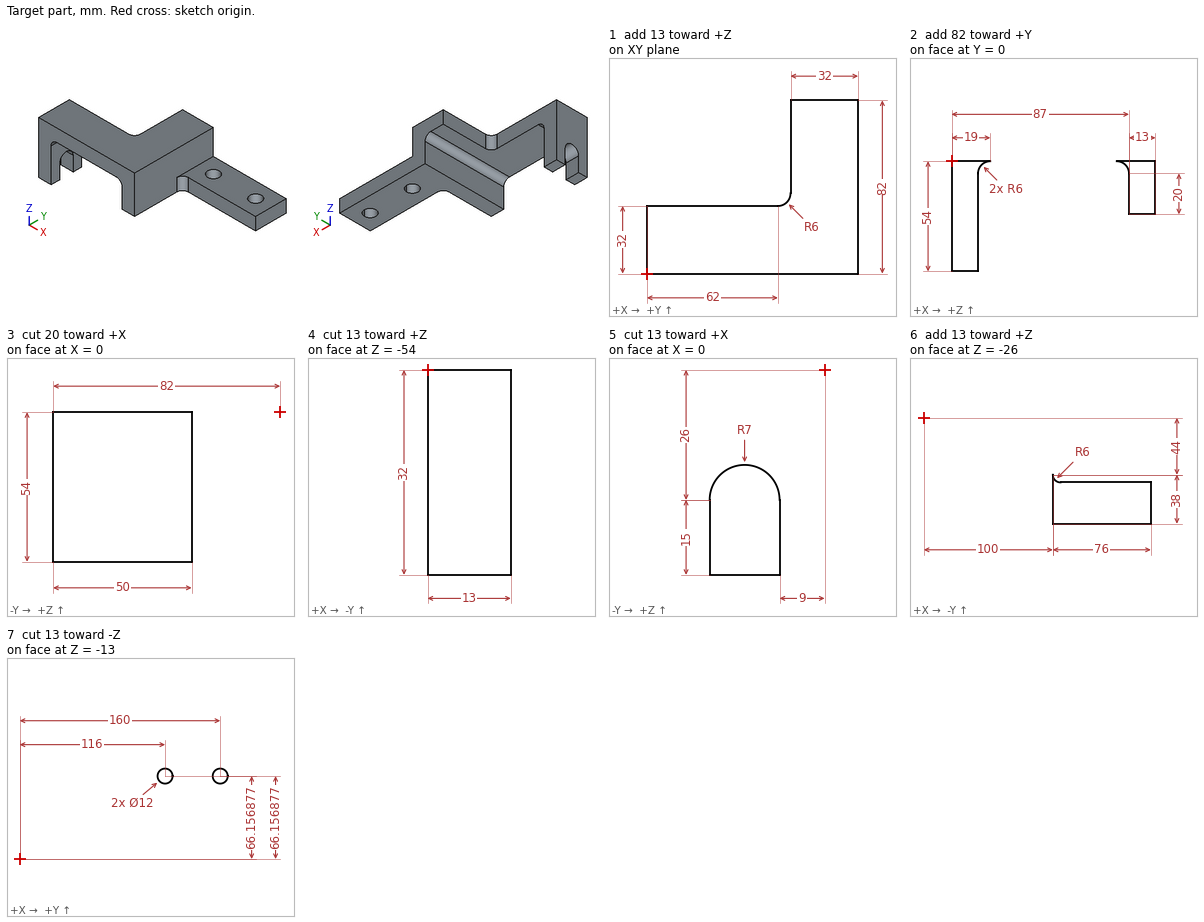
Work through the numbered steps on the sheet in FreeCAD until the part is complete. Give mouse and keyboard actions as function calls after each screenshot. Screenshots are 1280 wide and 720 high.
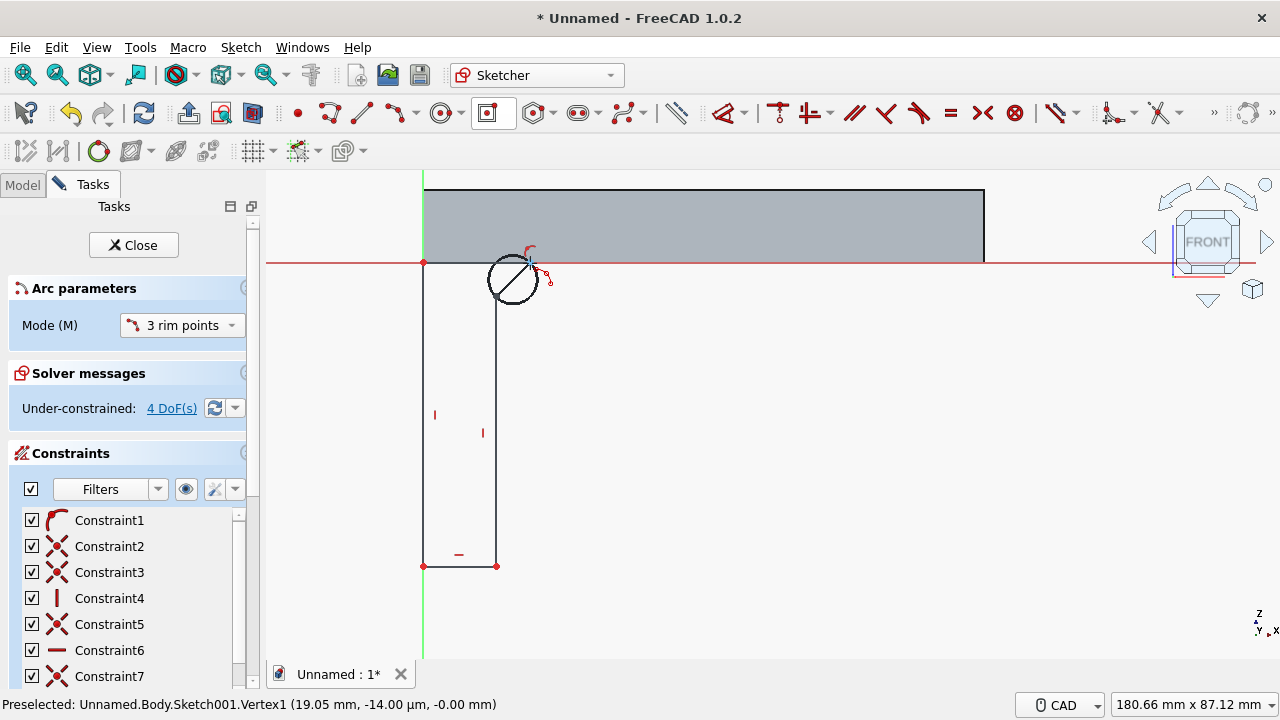
scroll(506, 272, up, 3)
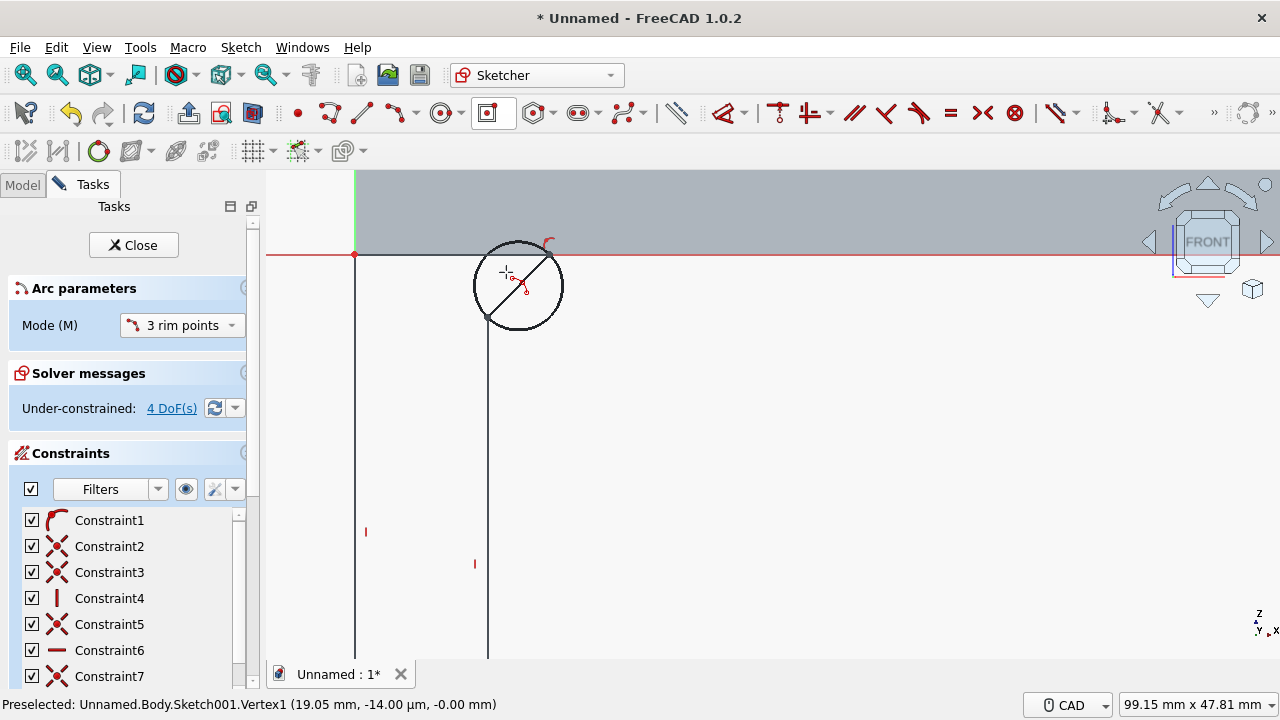
click(506, 273)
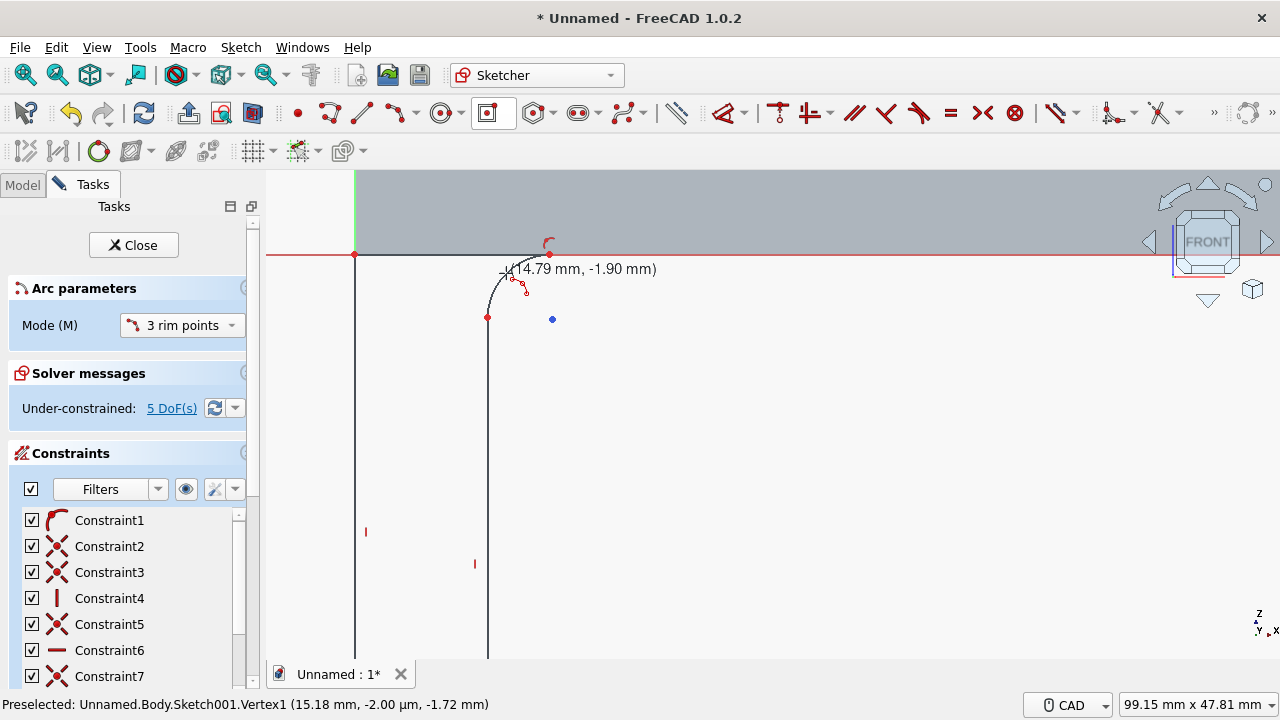
click(330, 114)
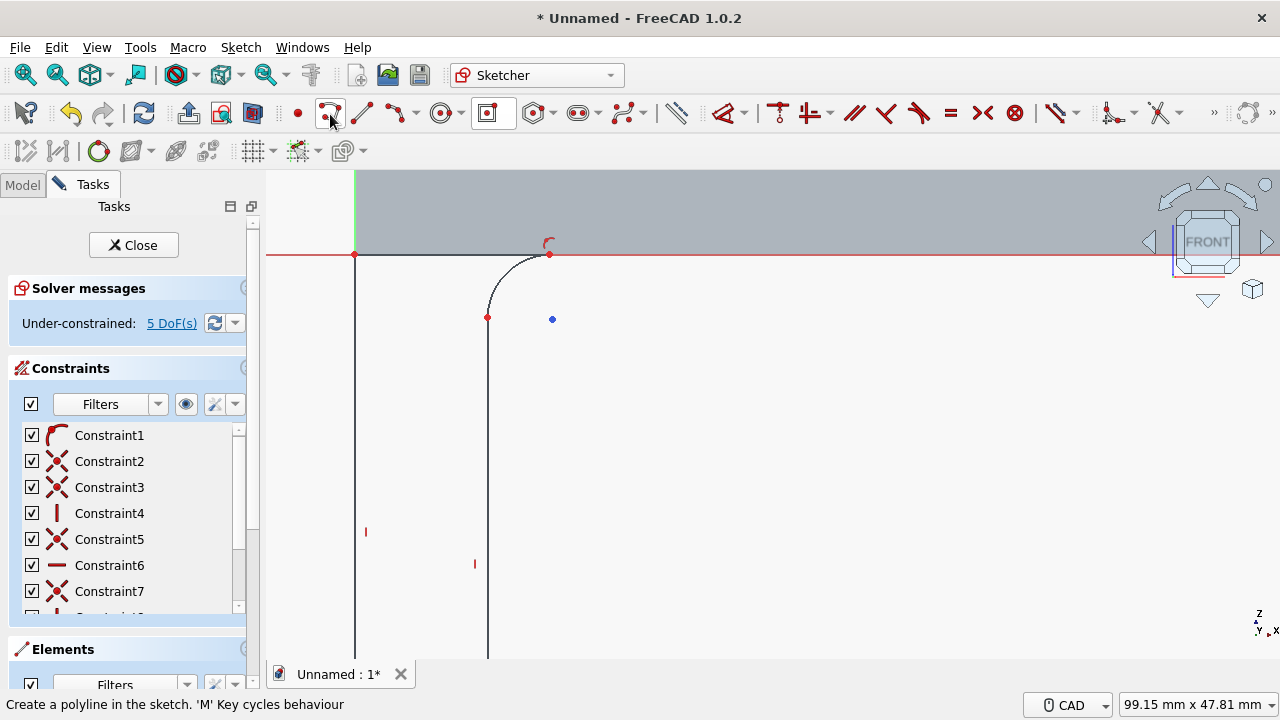
scroll(508, 273, down, 3)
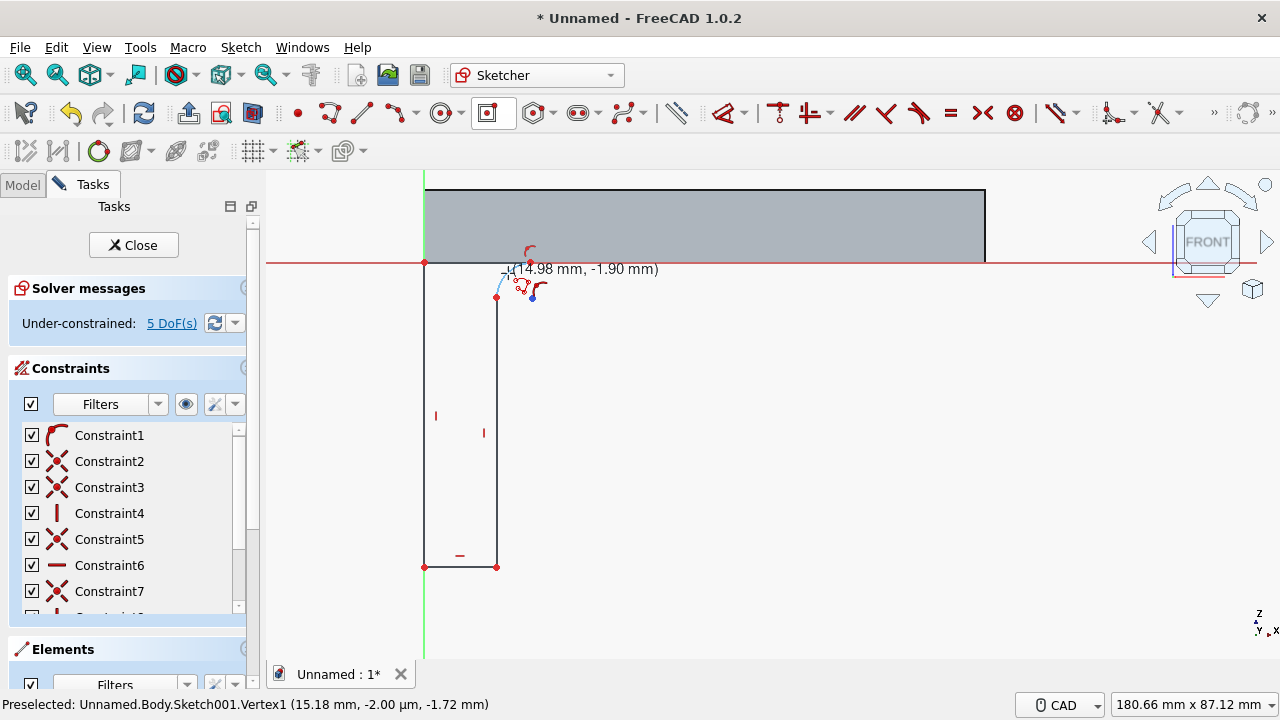
click(912, 297)
click(912, 409)
click(985, 409)
click(985, 263)
click(879, 272)
right_click(879, 272)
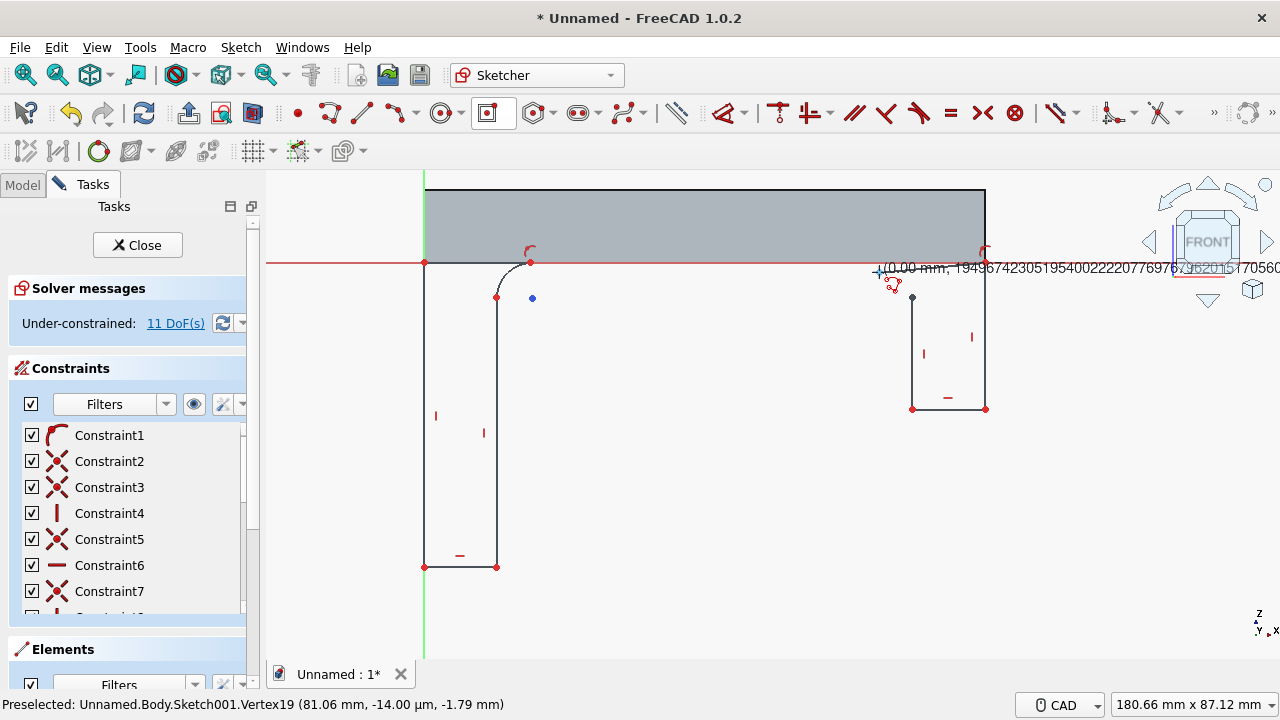
click(396, 114)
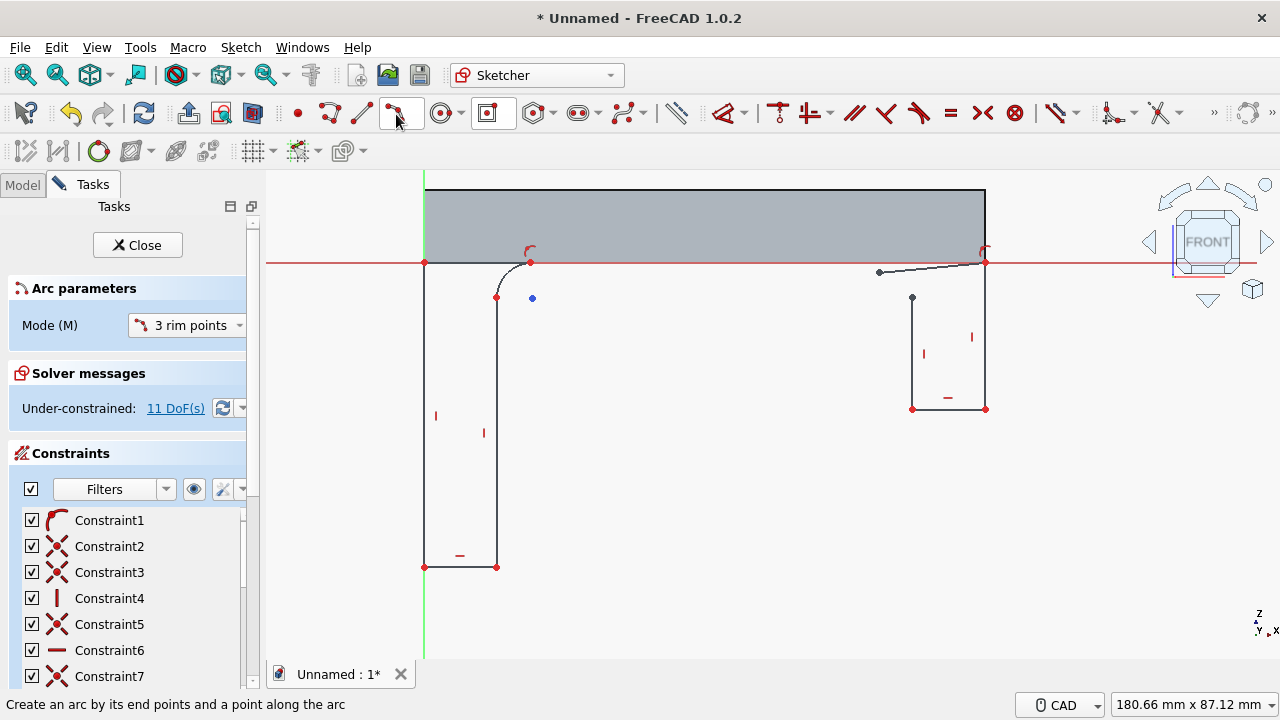
click(879, 273)
click(912, 298)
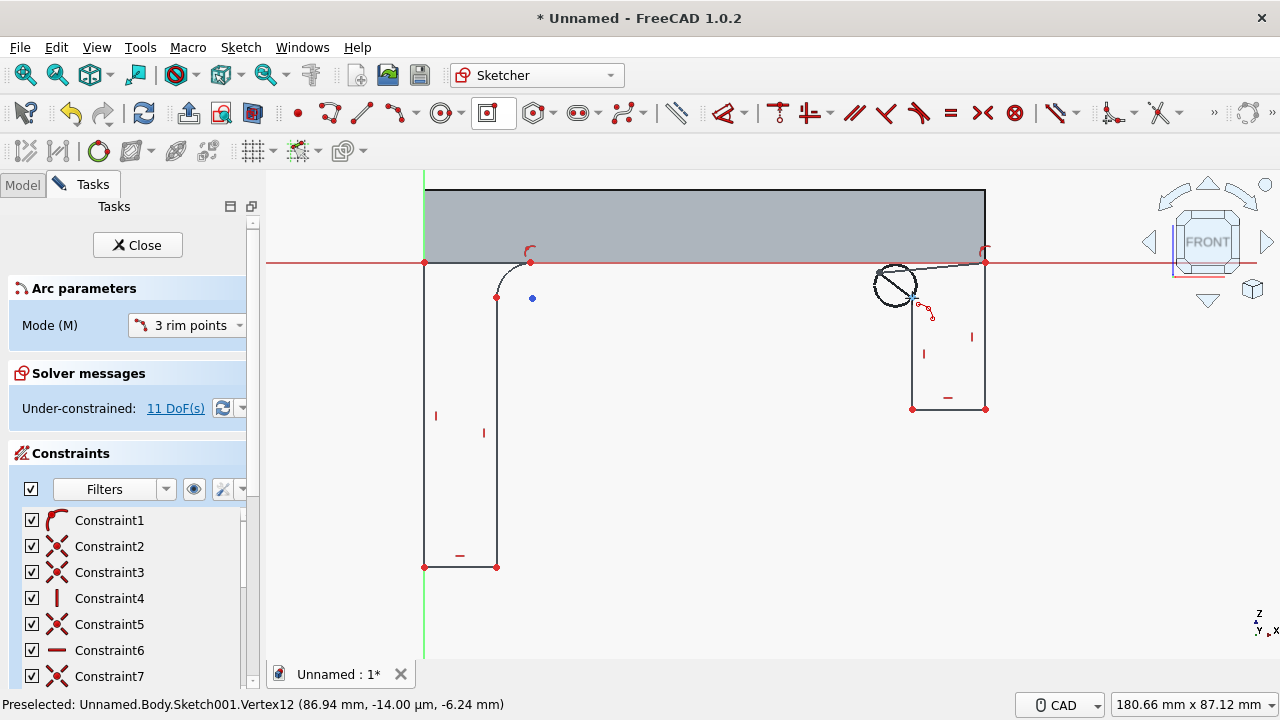
scroll(902, 273, up, 3)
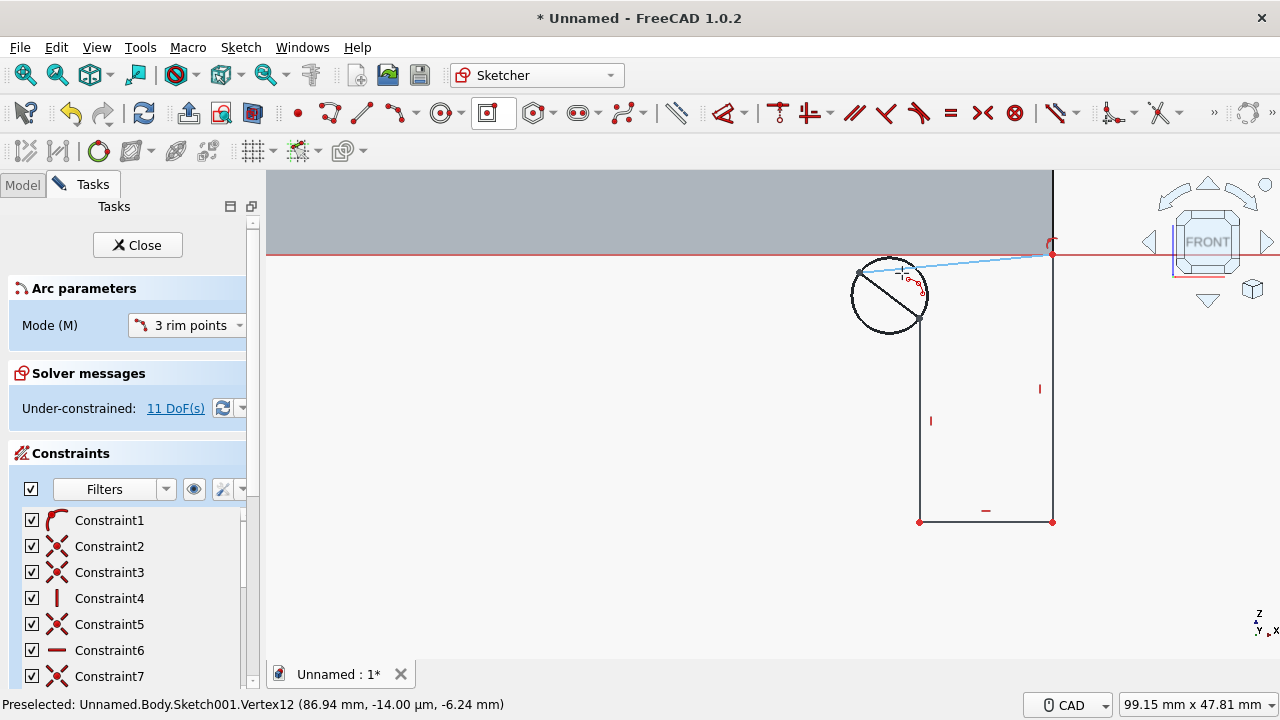
click(902, 273)
key(Escape)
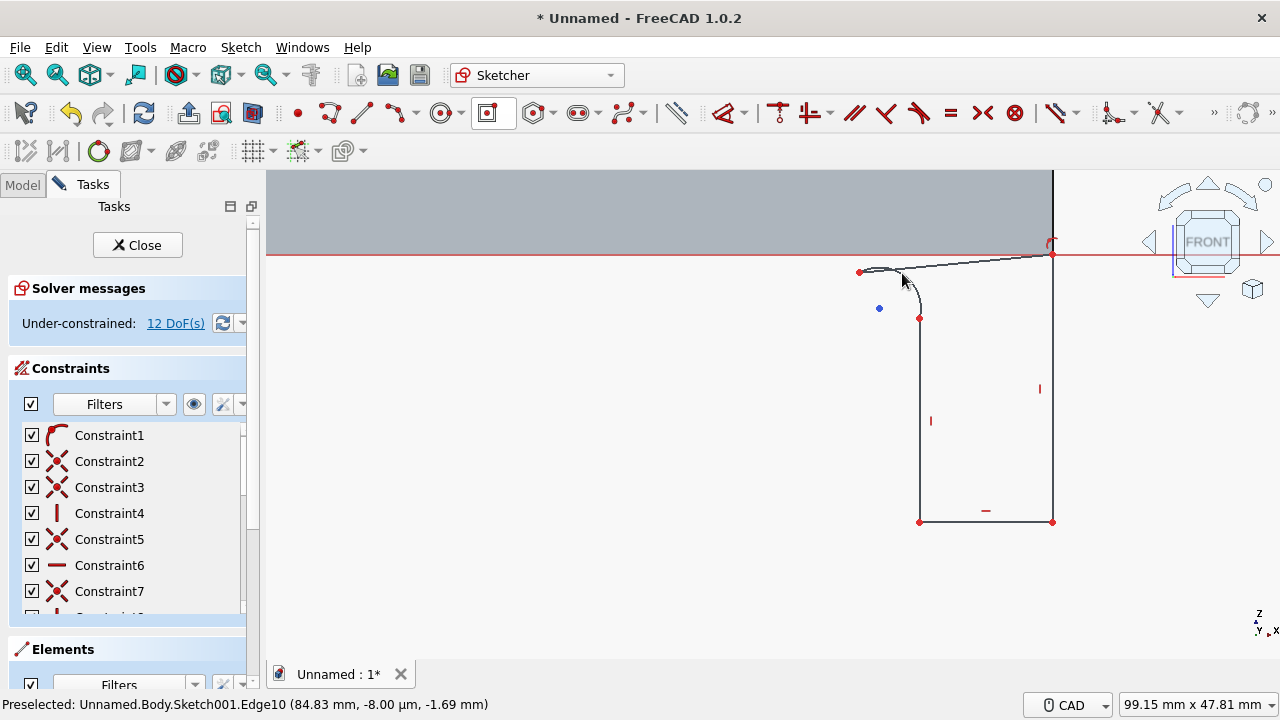
scroll(902, 273, down, 3)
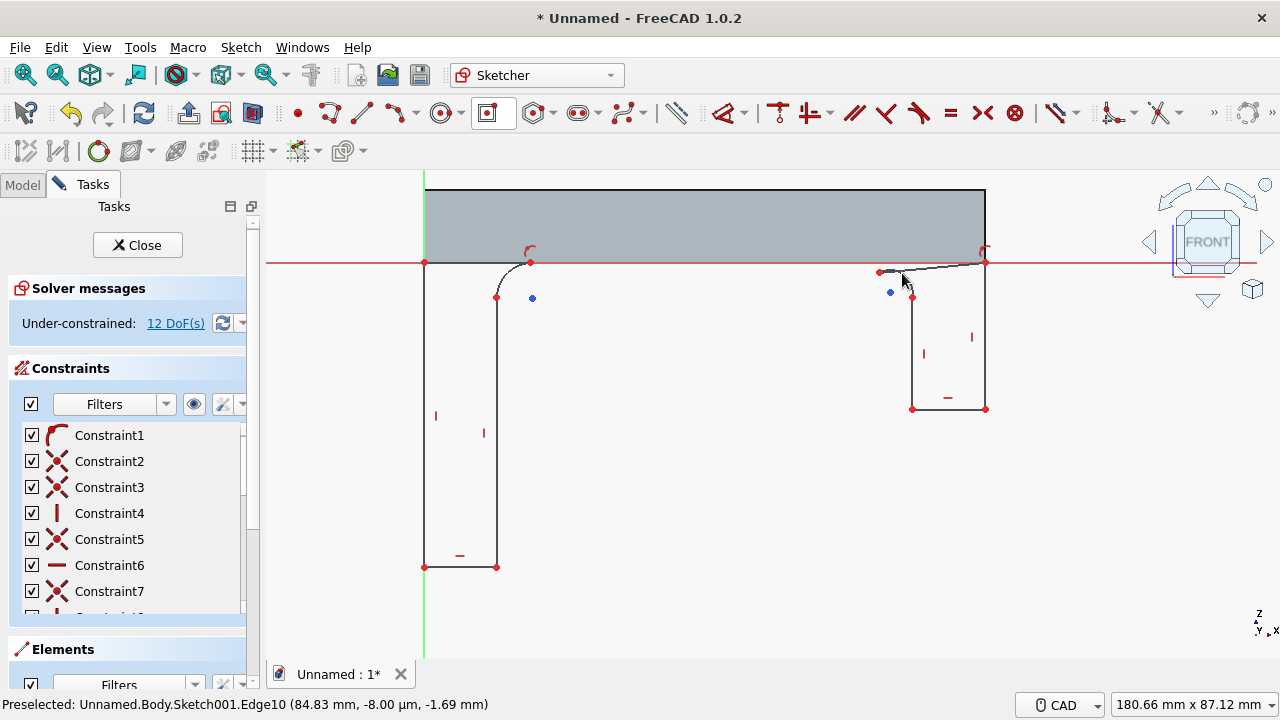
click(499, 263)